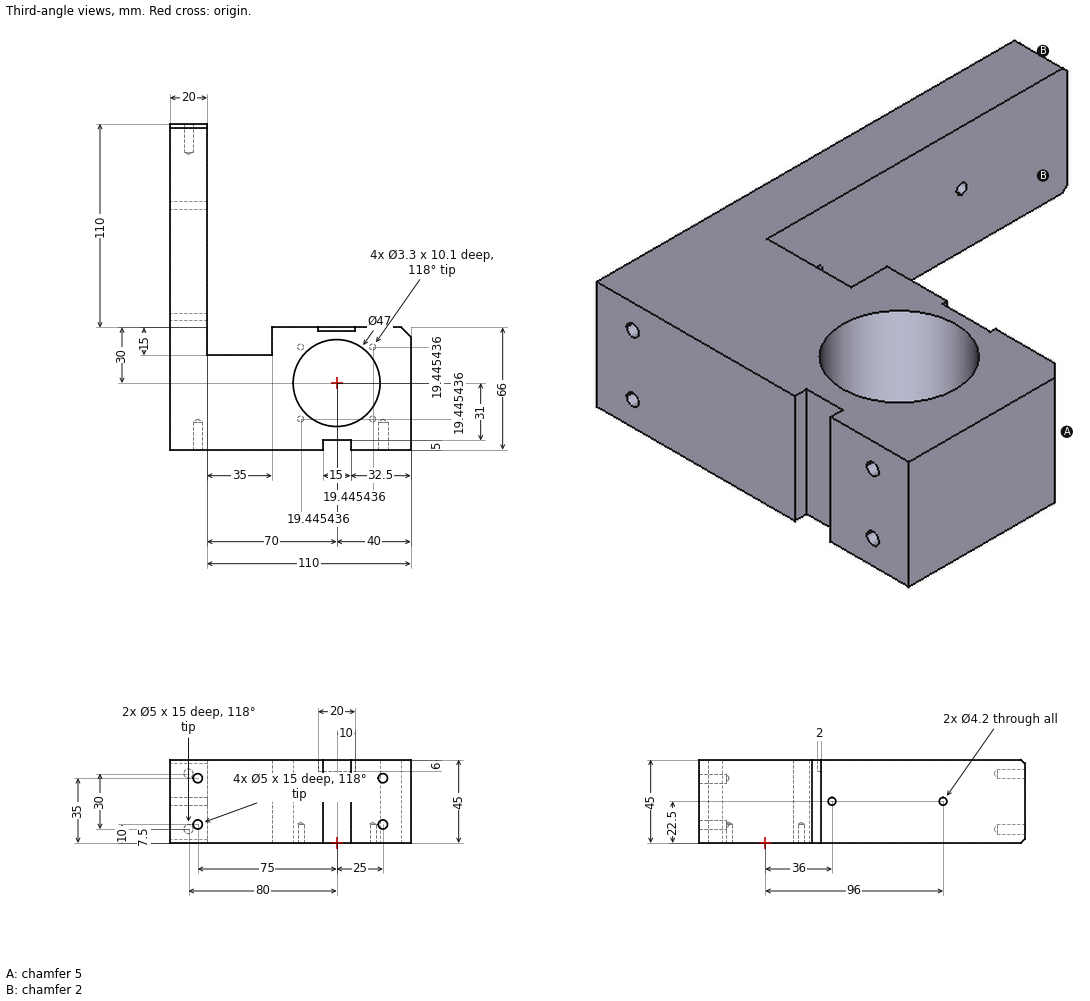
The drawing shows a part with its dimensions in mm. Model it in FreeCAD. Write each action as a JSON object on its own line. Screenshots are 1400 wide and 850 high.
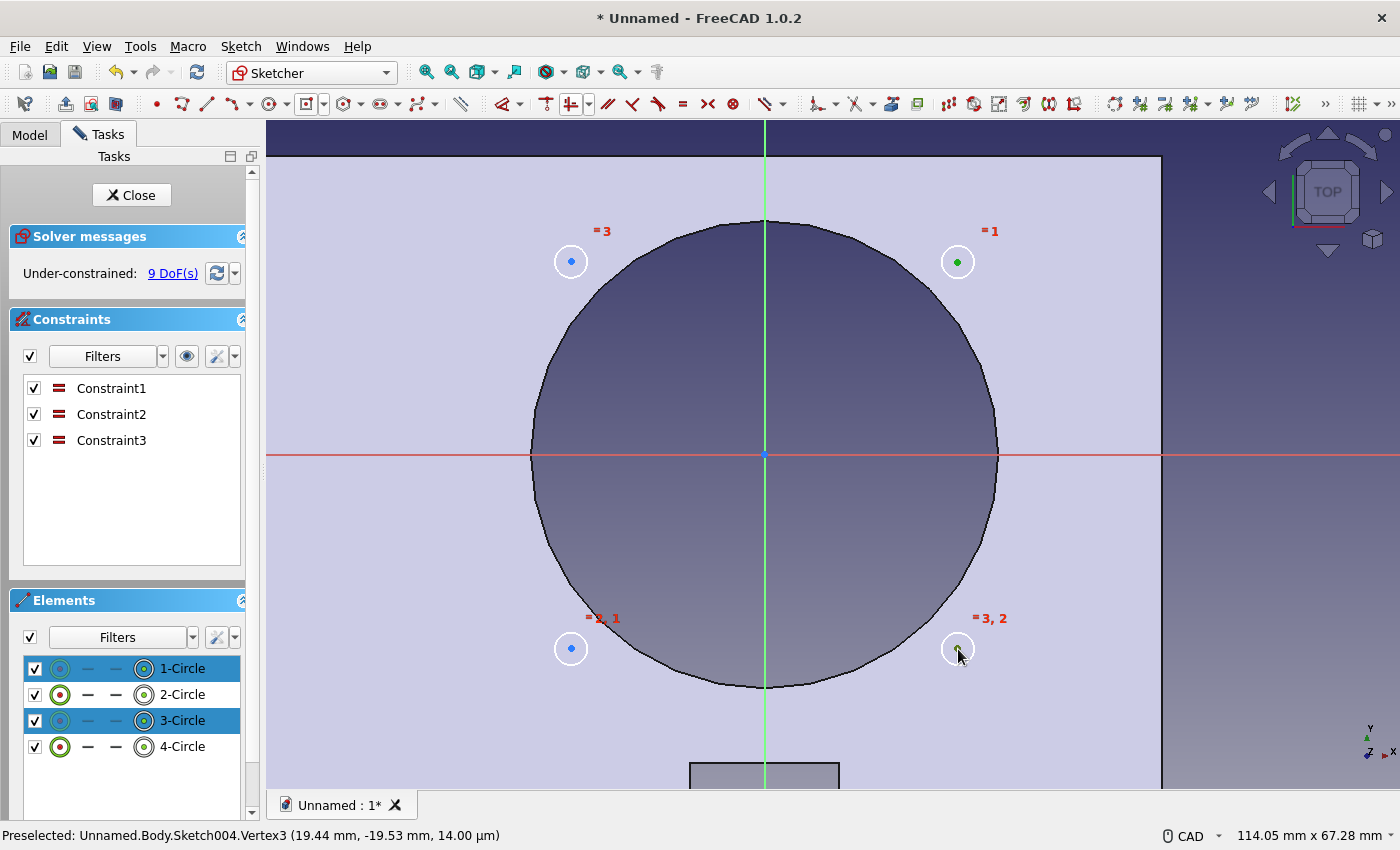
{"action": "key", "text": "v"}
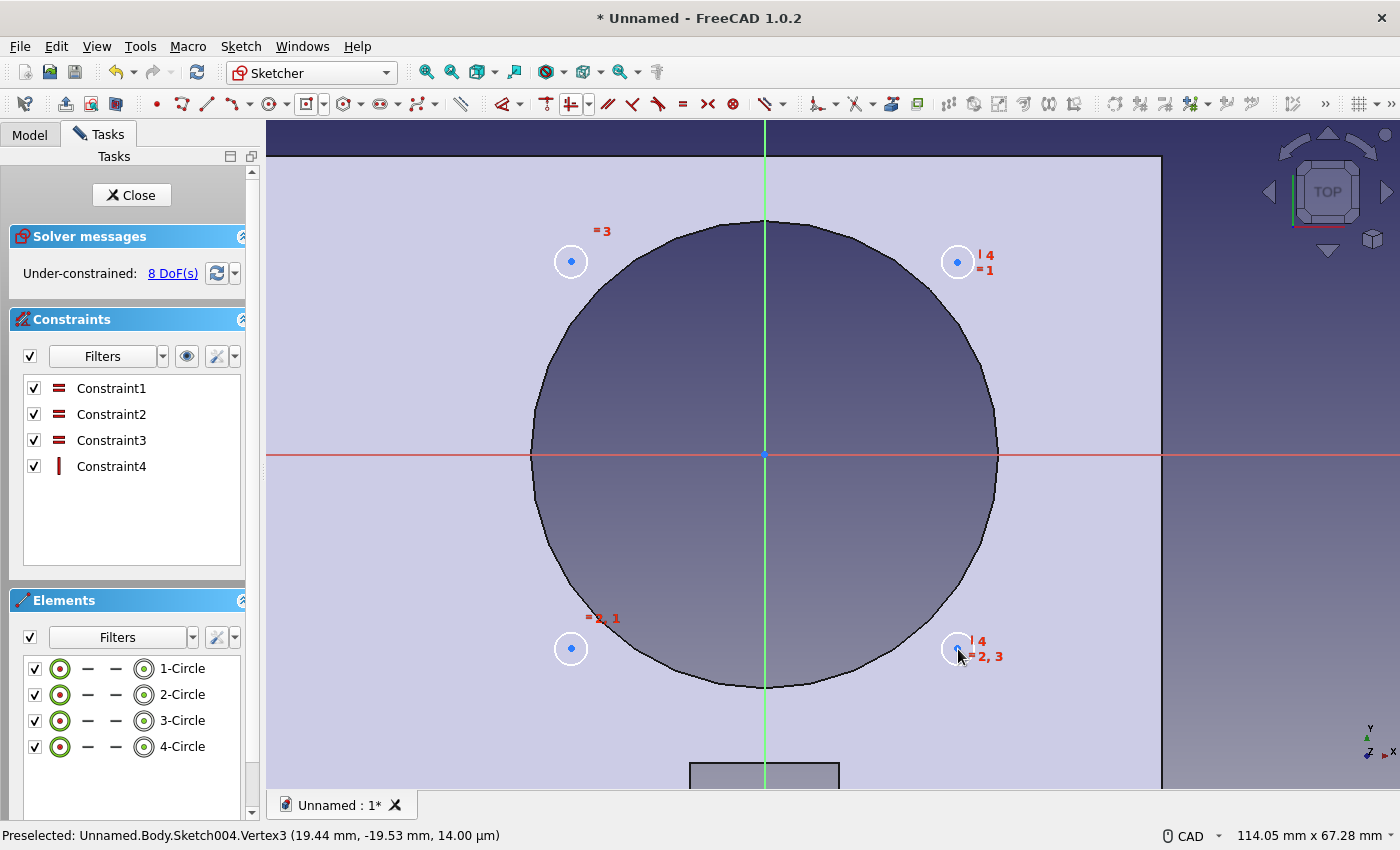
{"action": "left_click", "coordinate": [571, 649]}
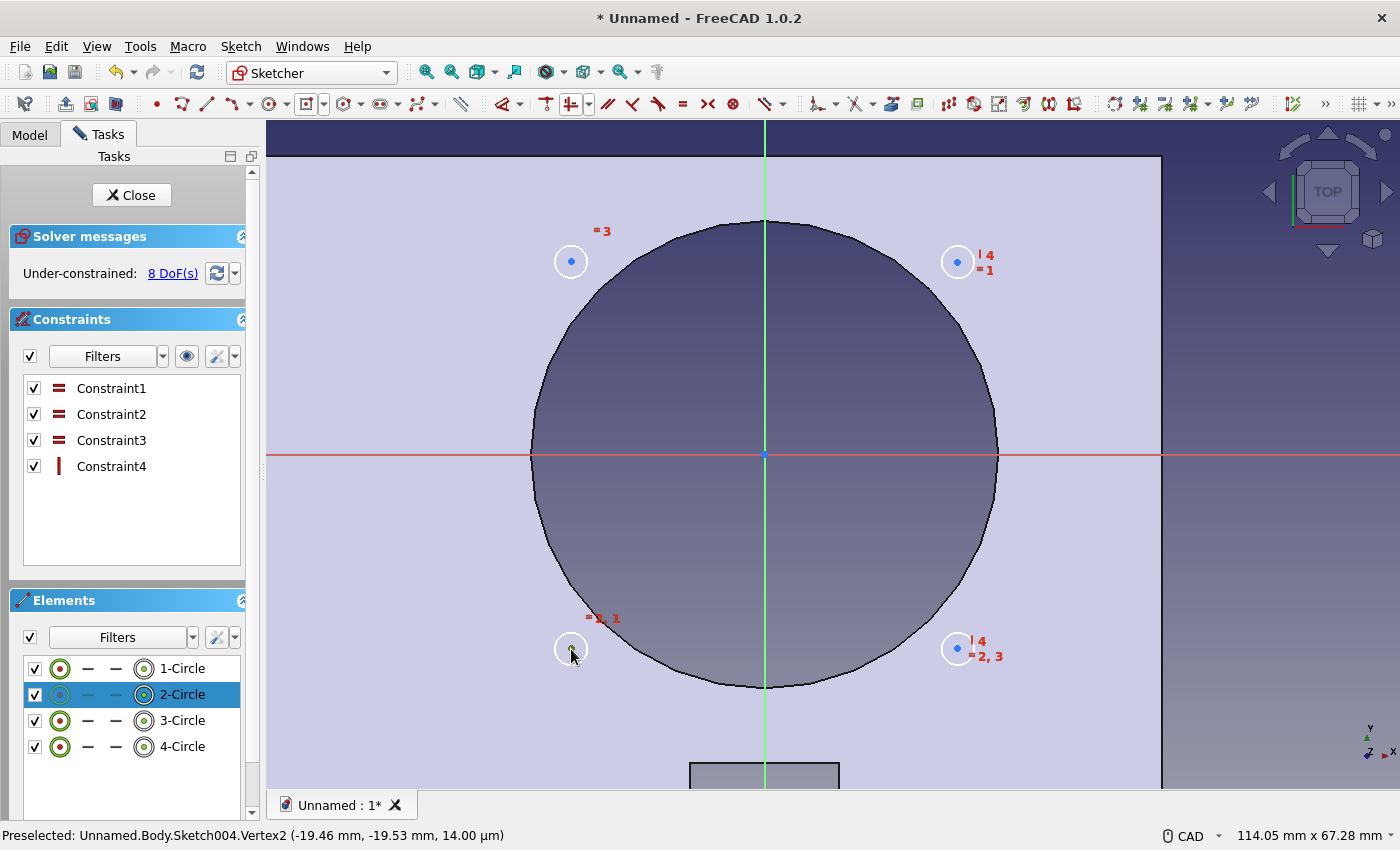
{"action": "left_click", "coordinate": [958, 649]}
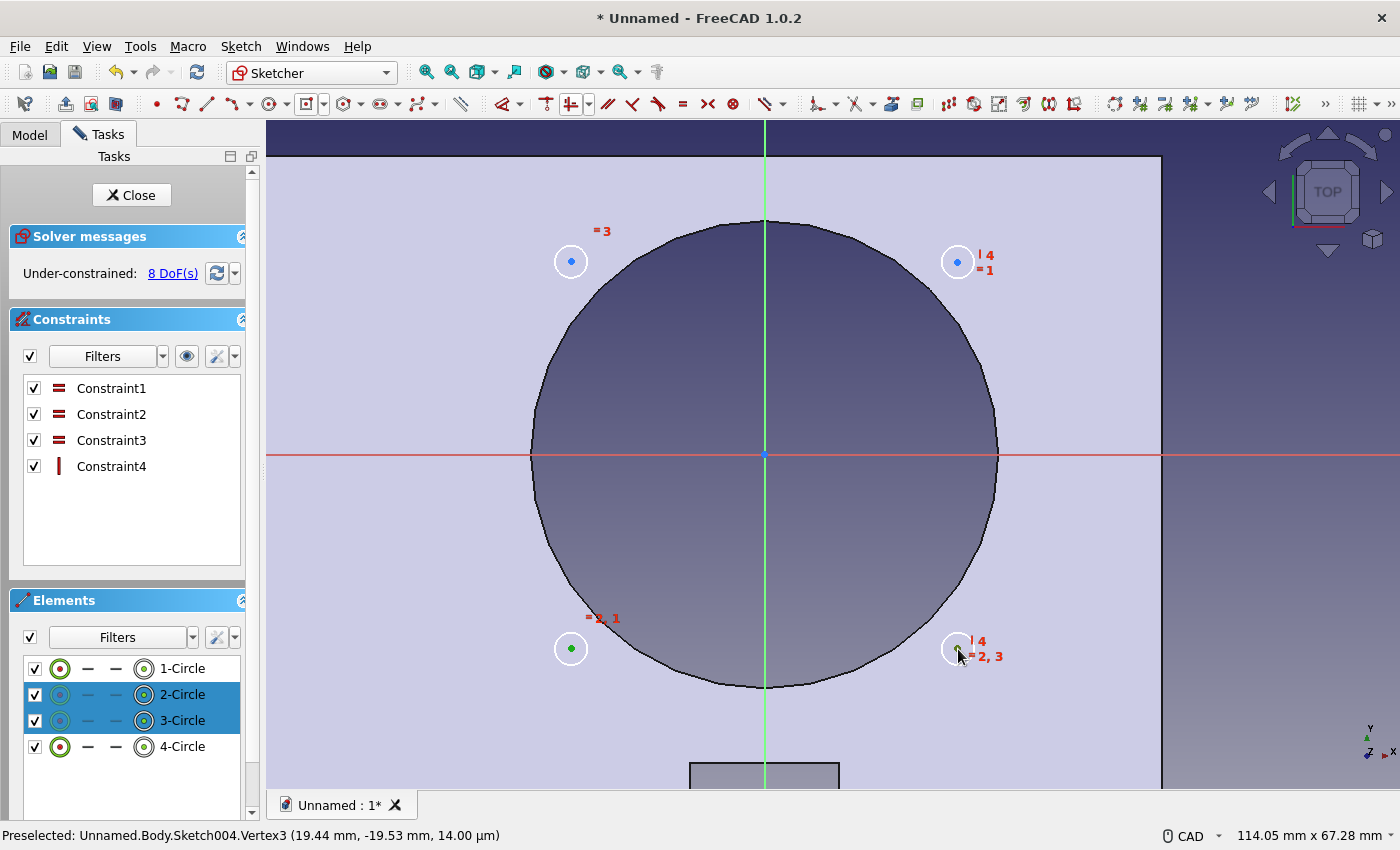
{"action": "left_click", "coordinate": [588, 104]}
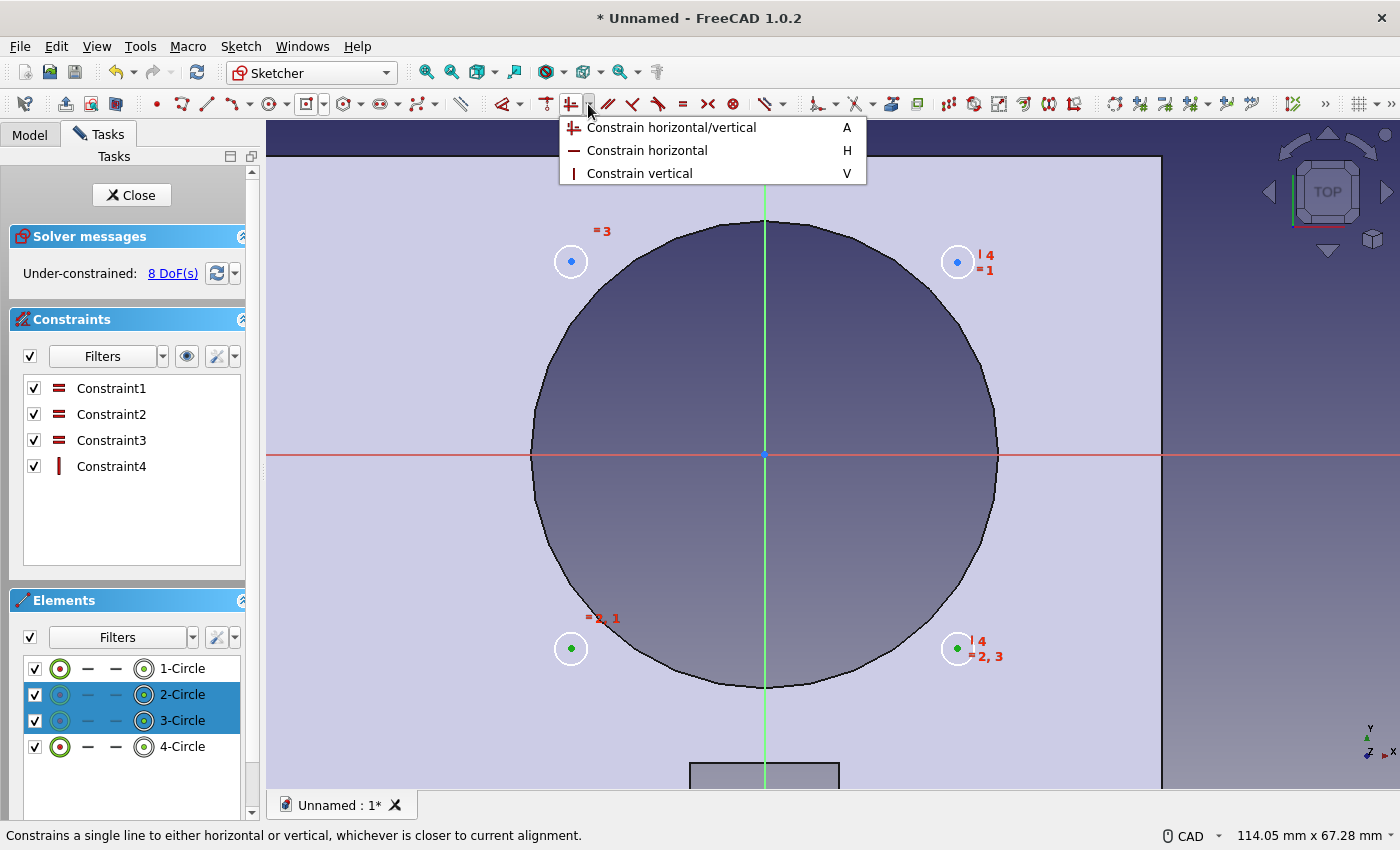
{"action": "left_click", "coordinate": [713, 150]}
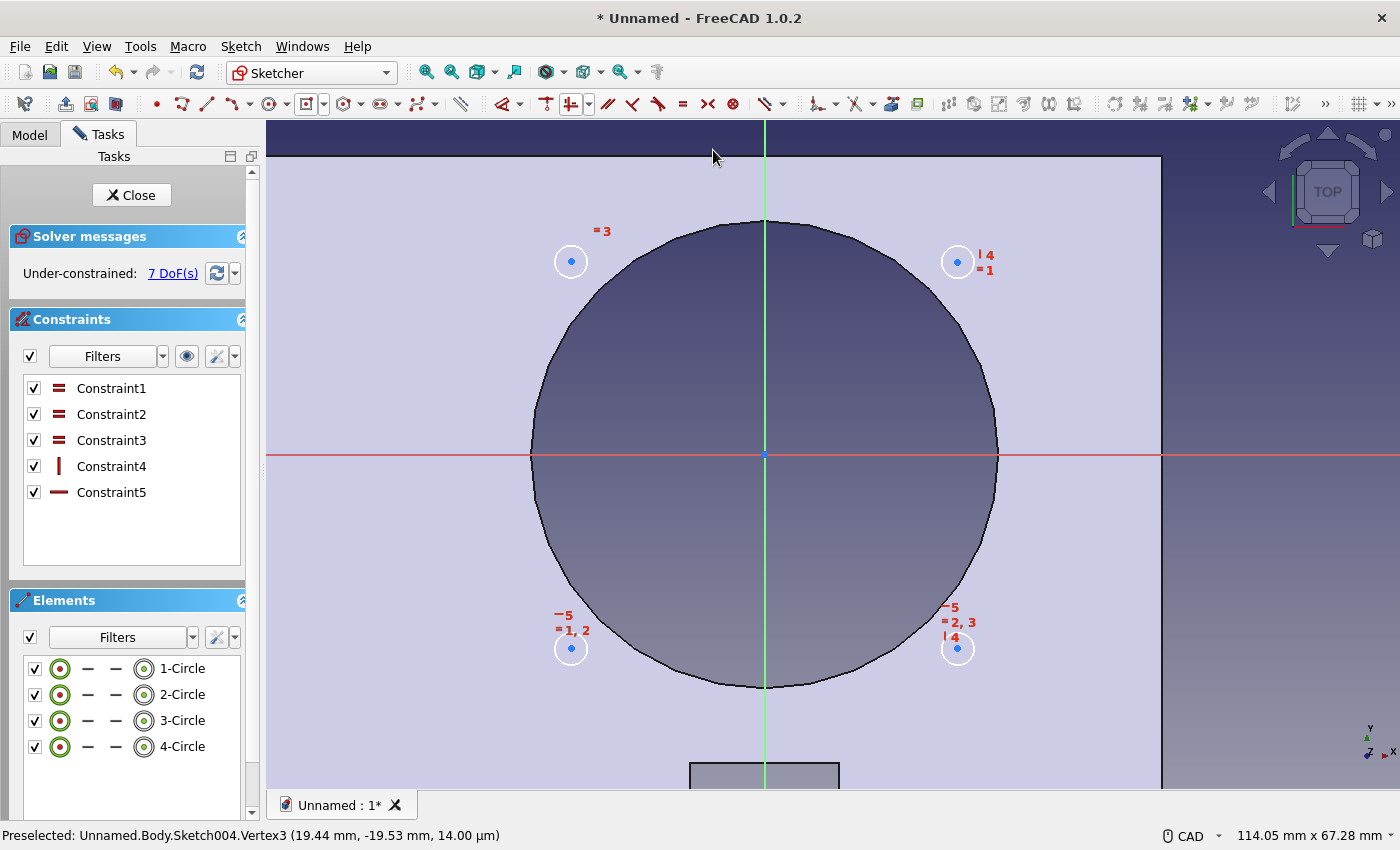
{"action": "left_click", "coordinate": [571, 649]}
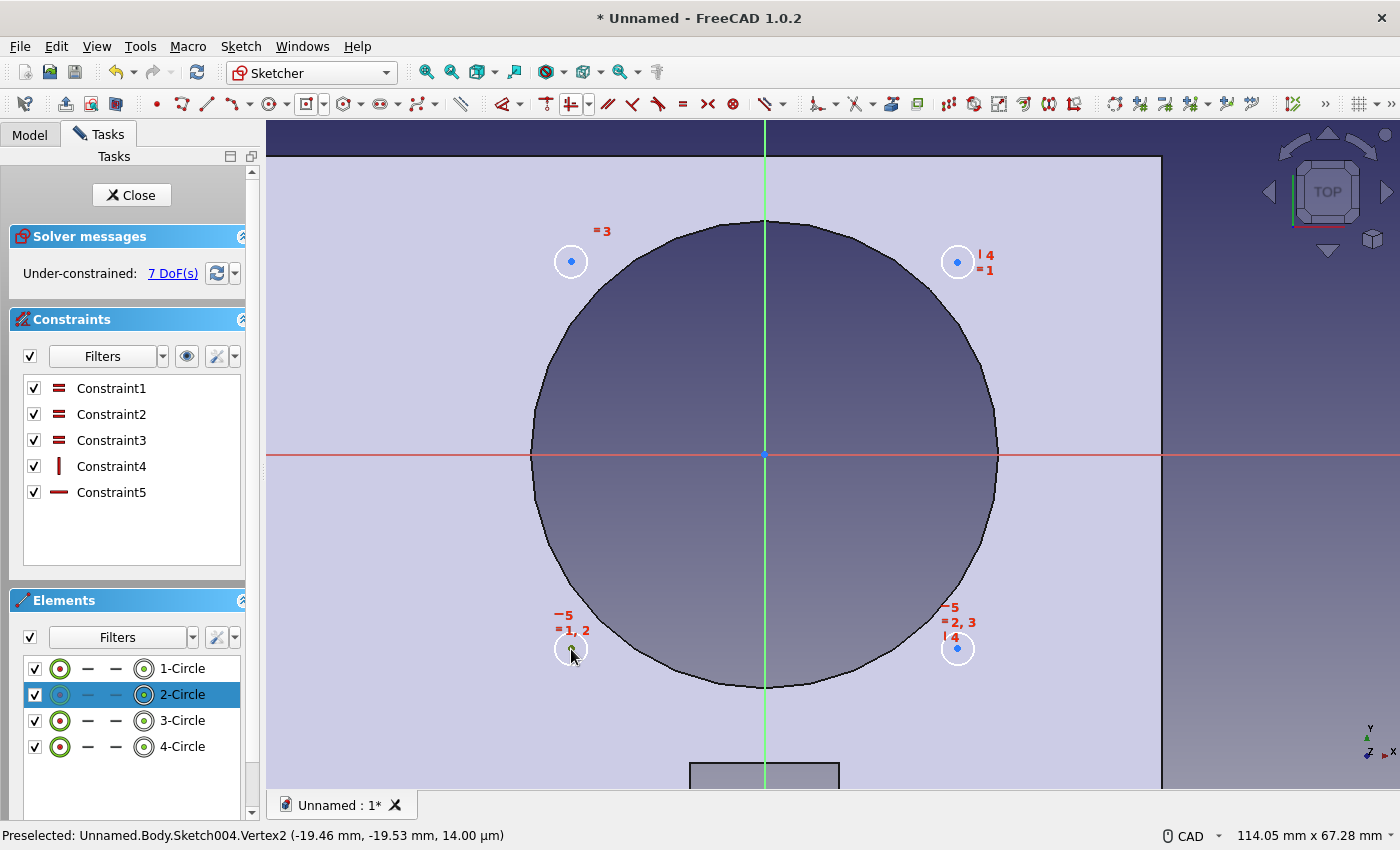
{"action": "left_click", "coordinate": [571, 262]}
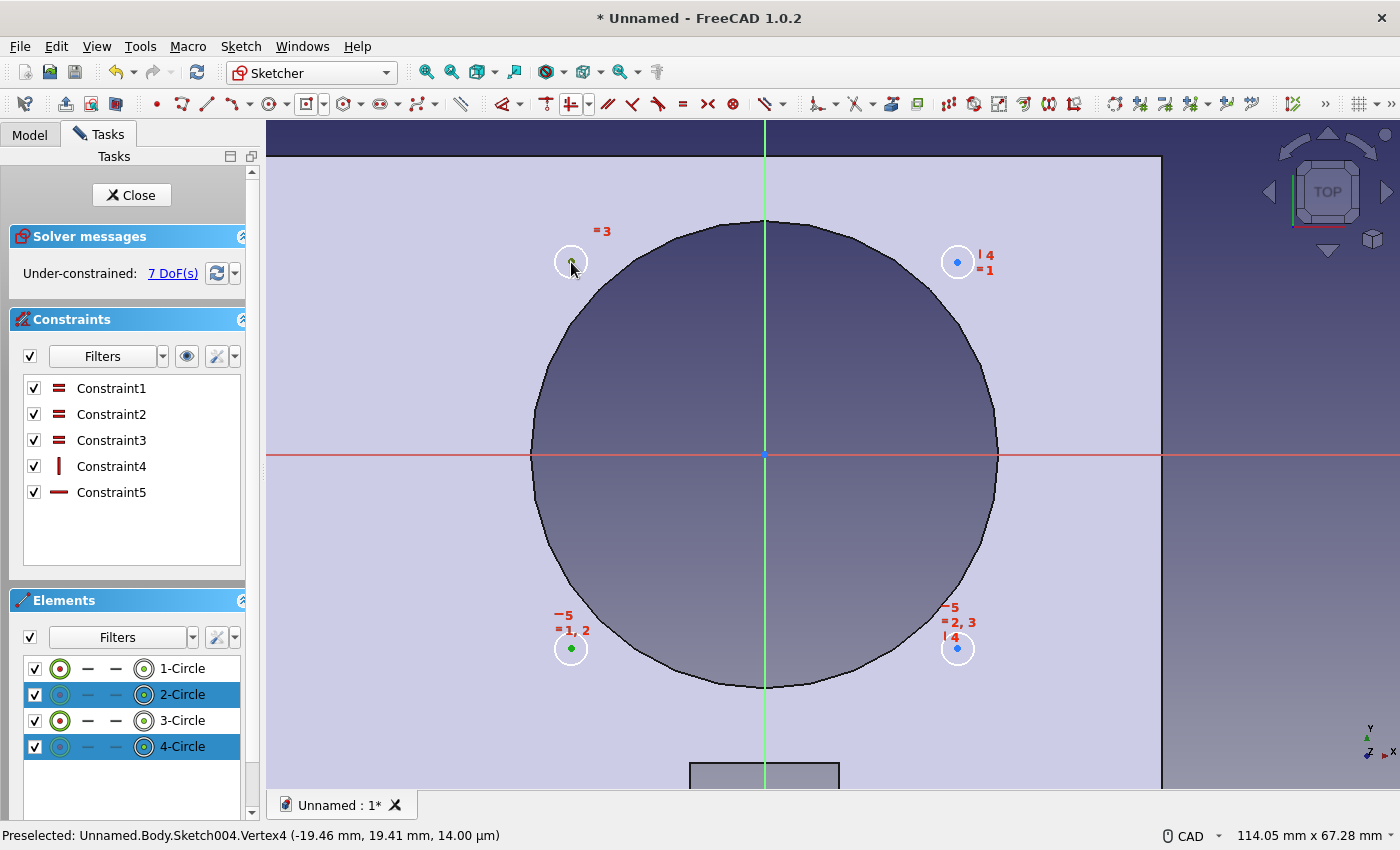
{"action": "key", "text": "v"}